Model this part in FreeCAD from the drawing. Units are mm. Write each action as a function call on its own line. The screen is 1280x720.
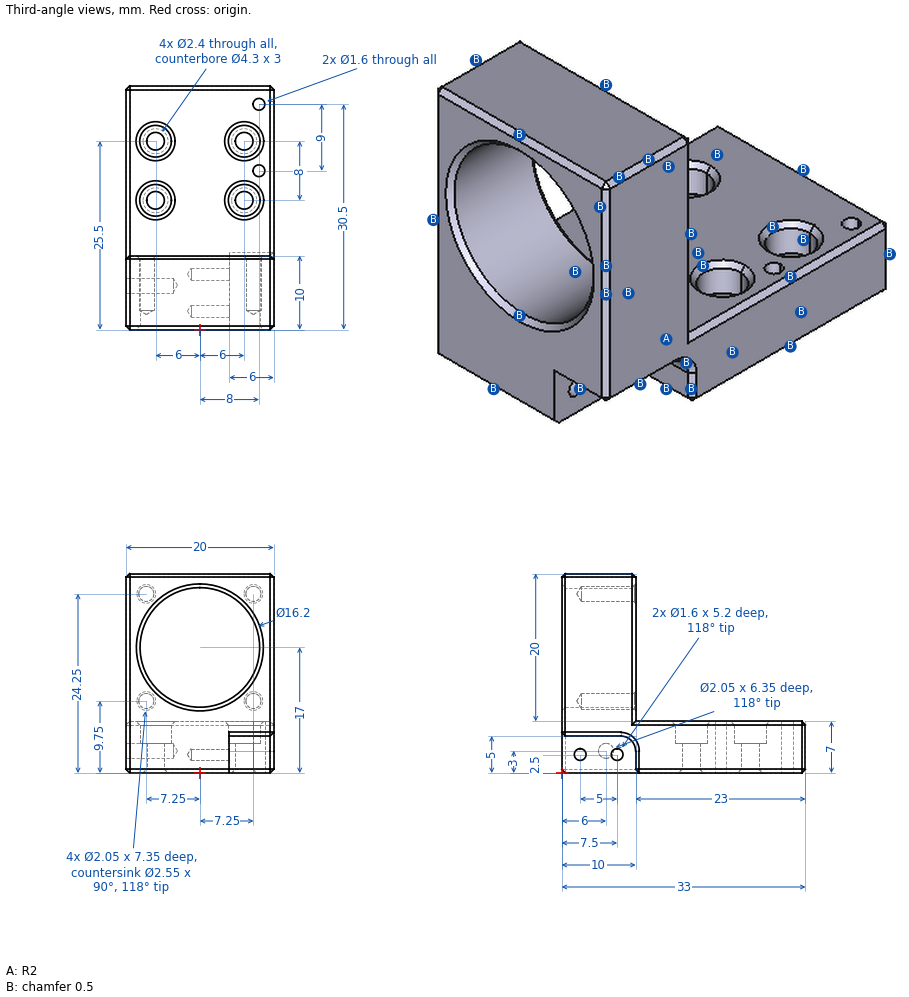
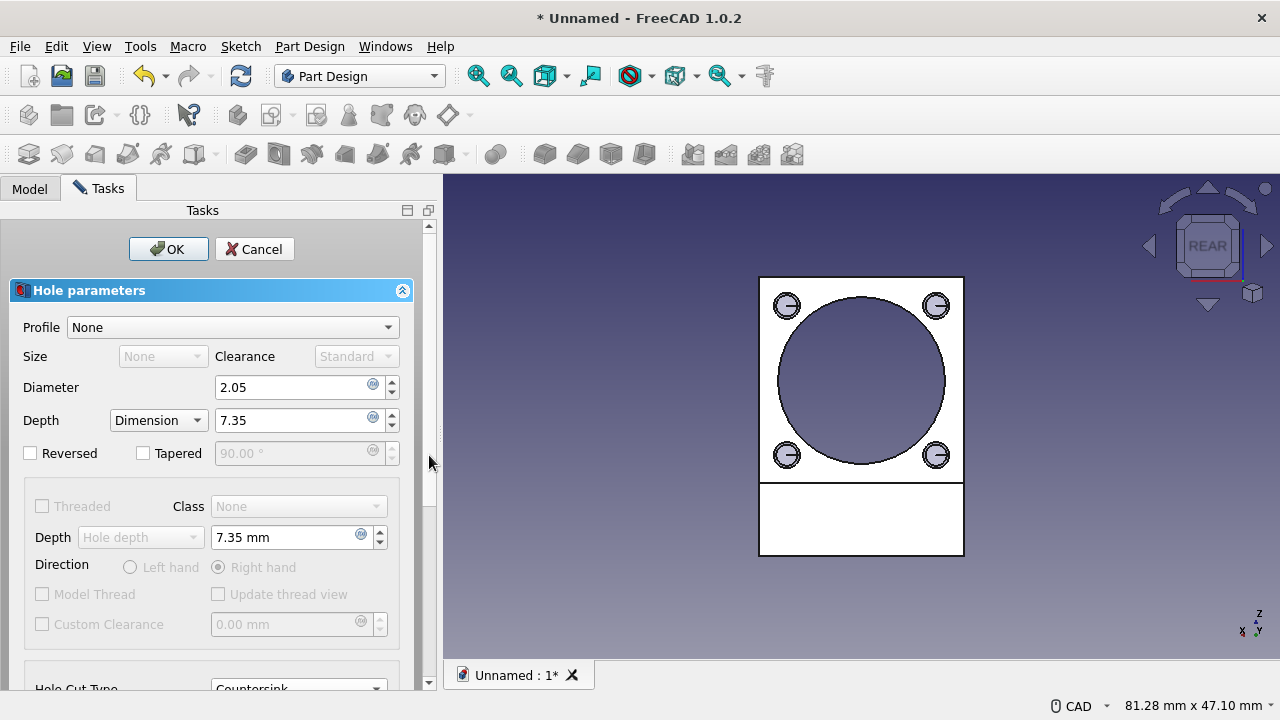
click(169, 249)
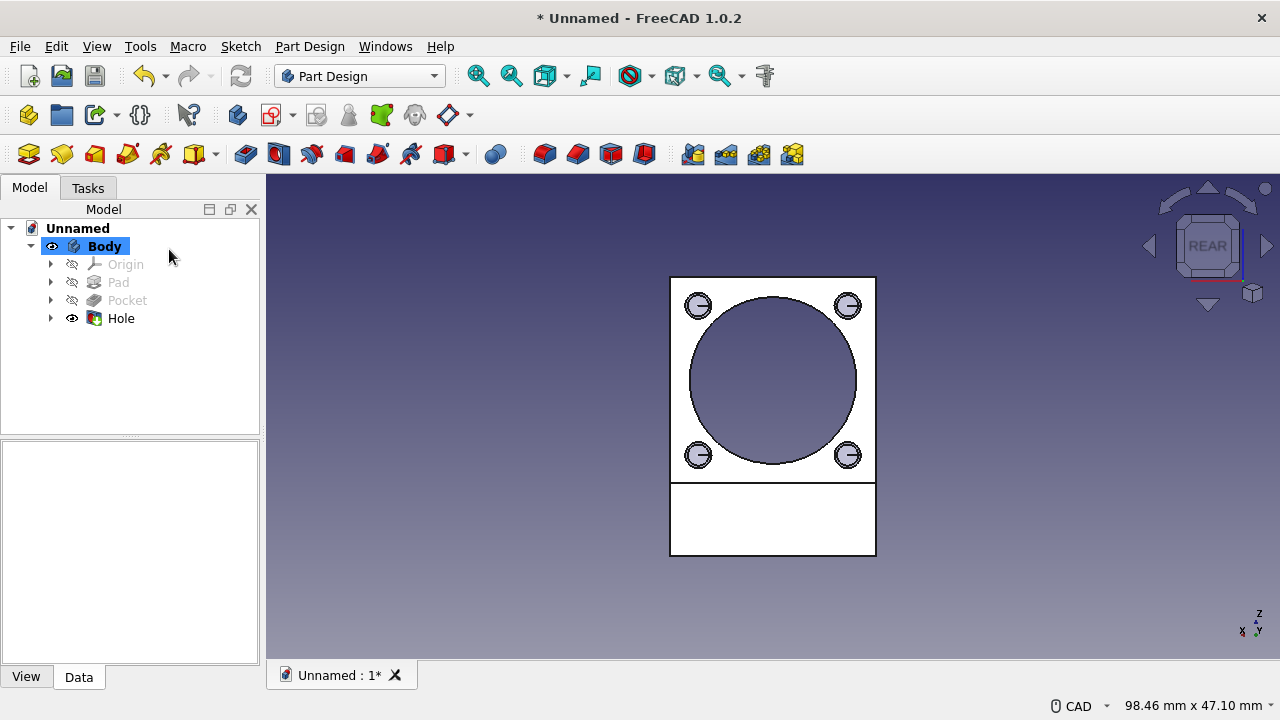
key(0)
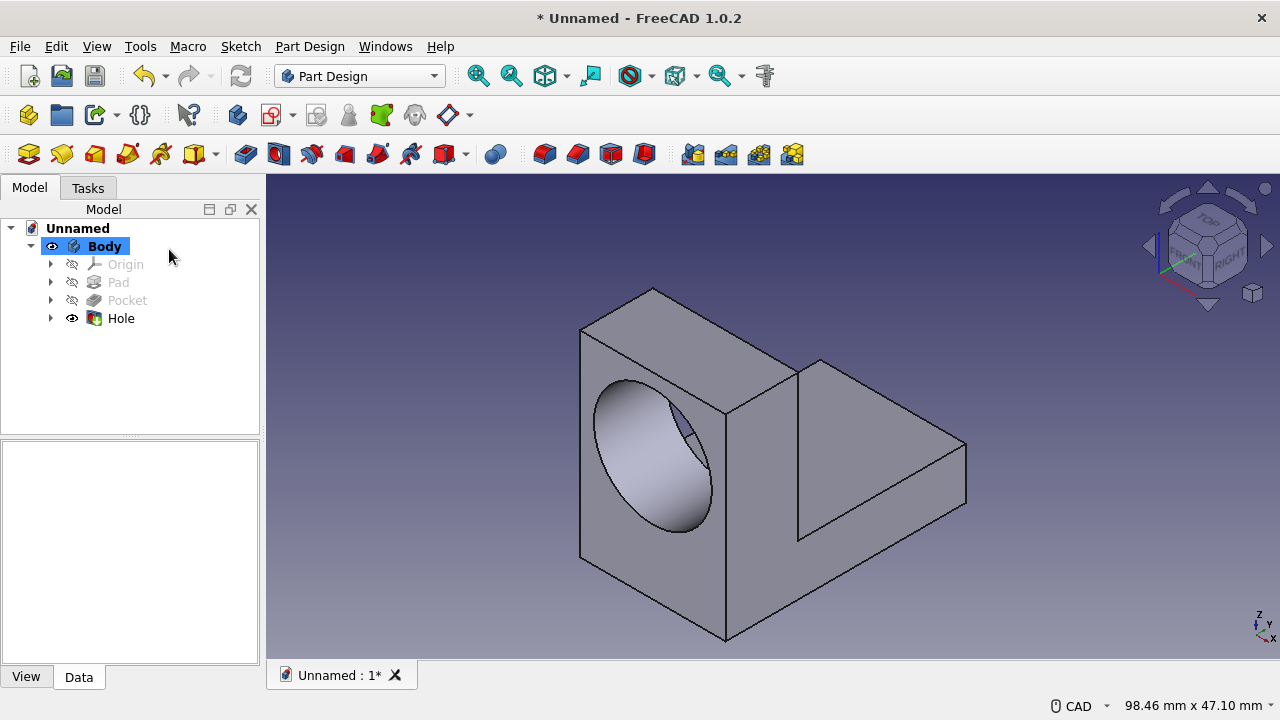
click(809, 449)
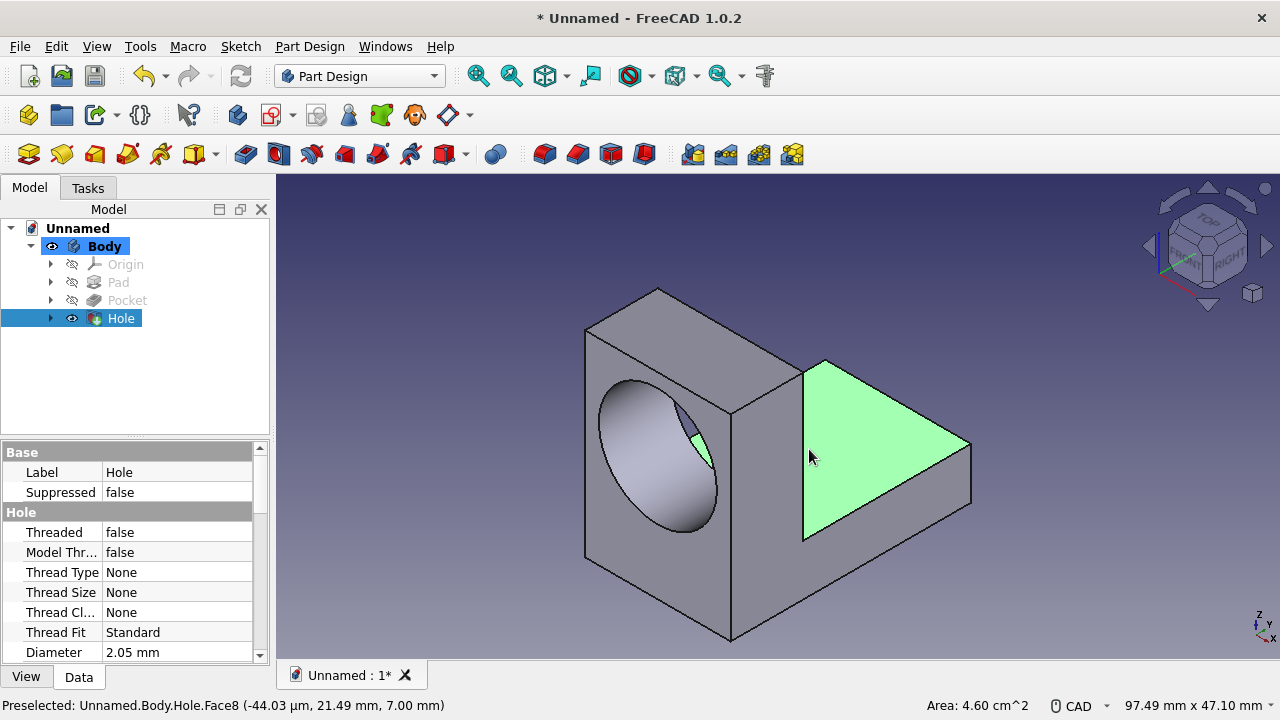
click(270, 116)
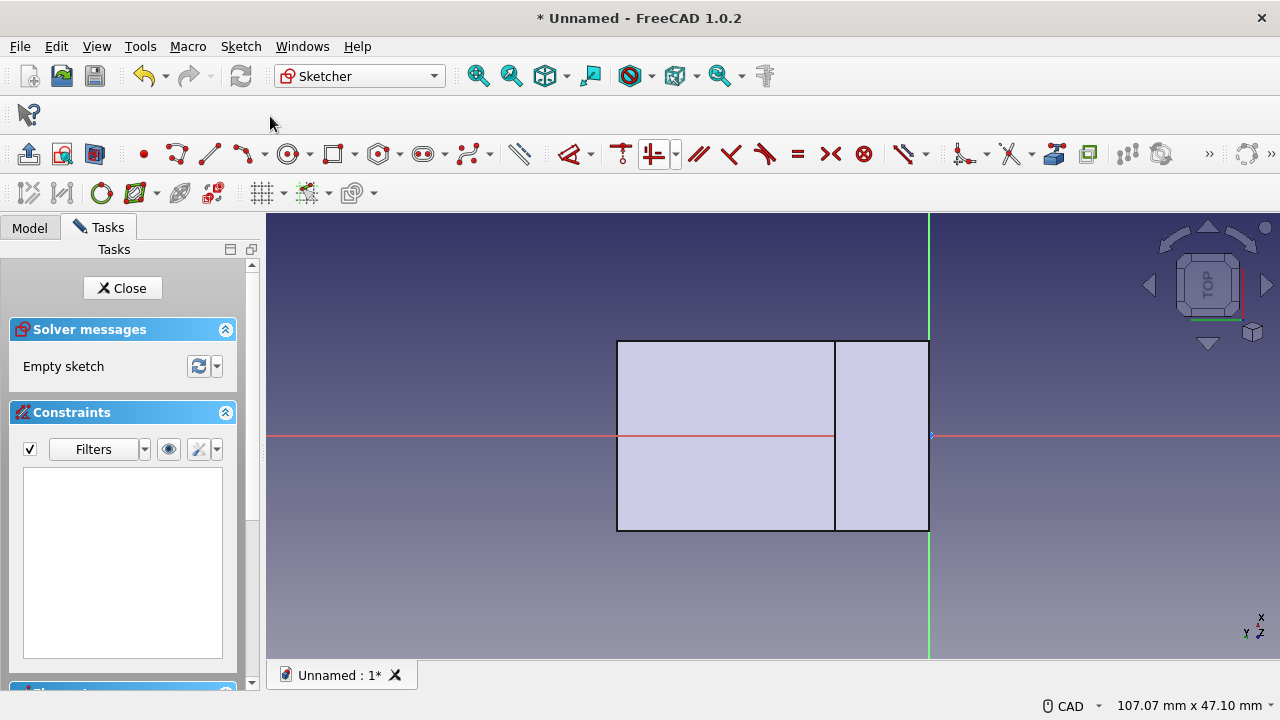
scroll(883, 436, up, 4)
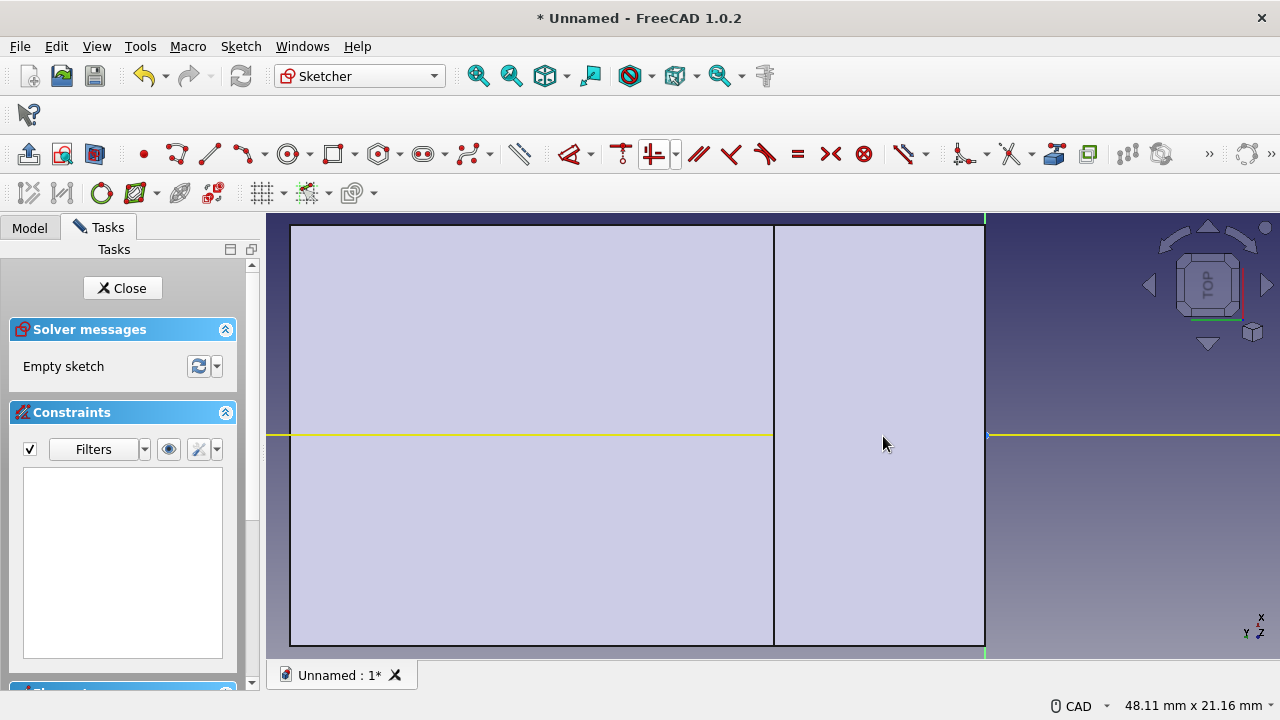
key(g)
key(c)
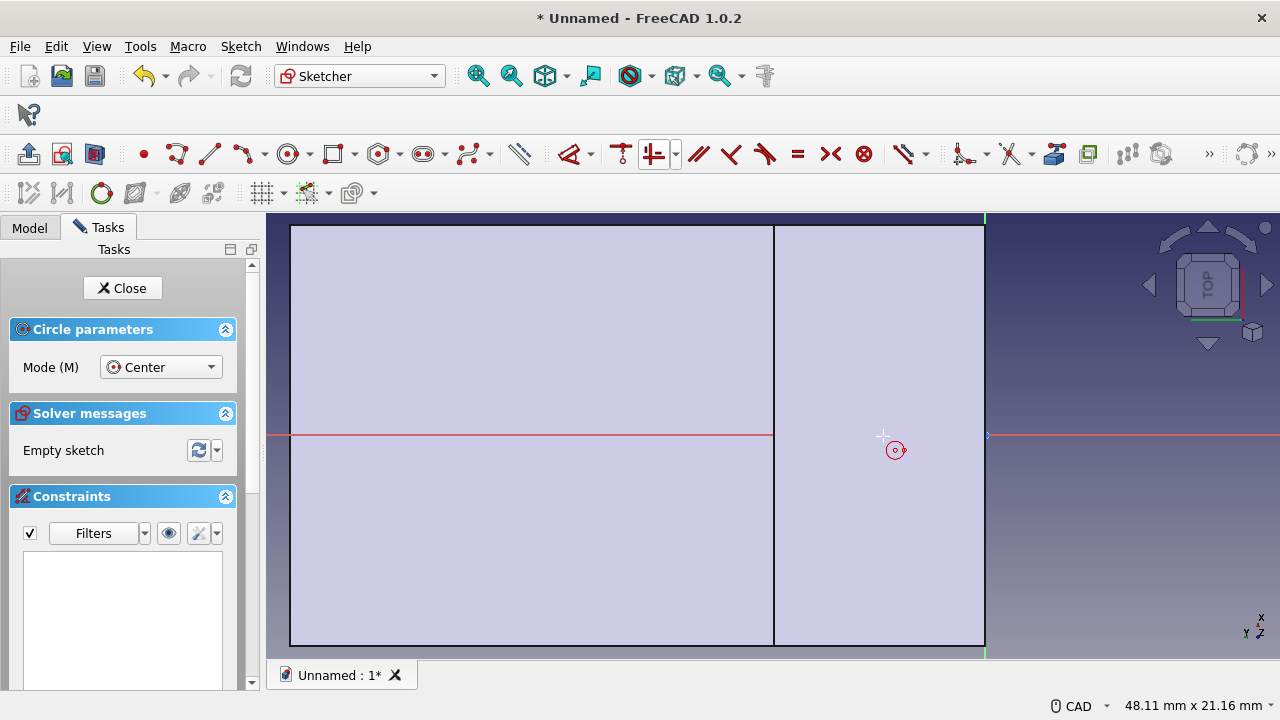
click(448, 562)
move(466, 544)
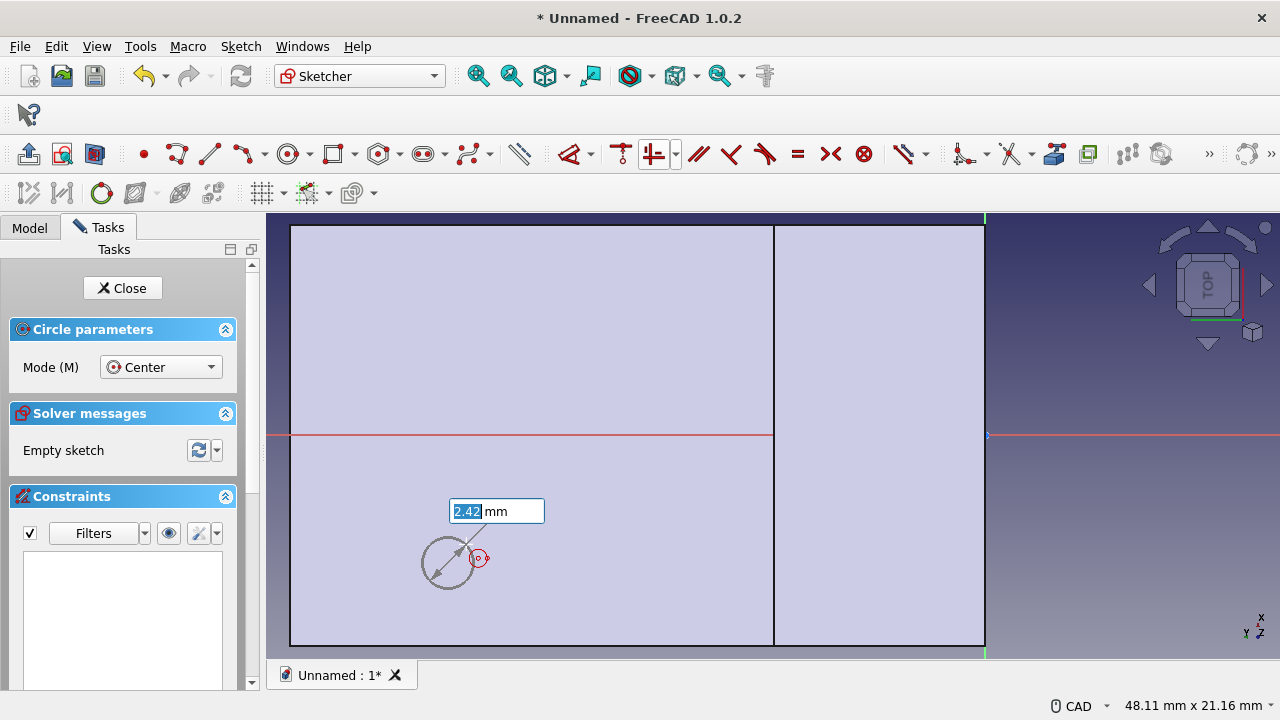
text(2.4)
key(Return)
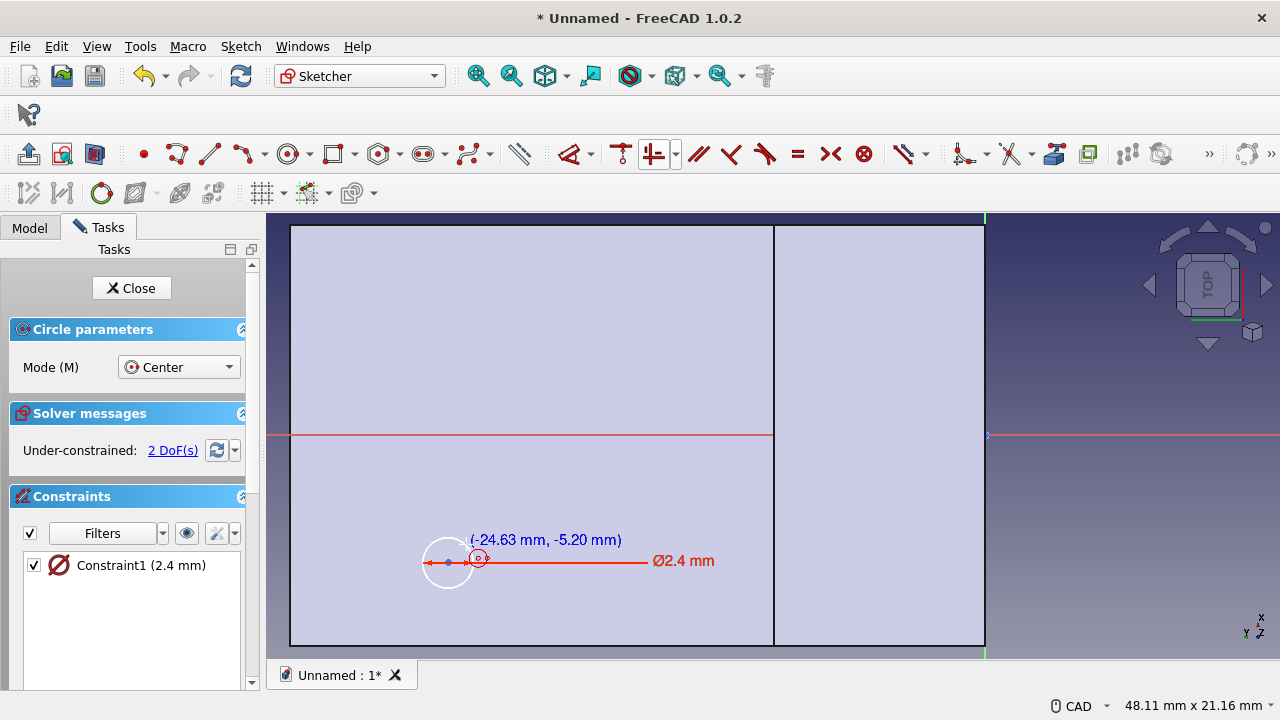
click(448, 309)
move(466, 291)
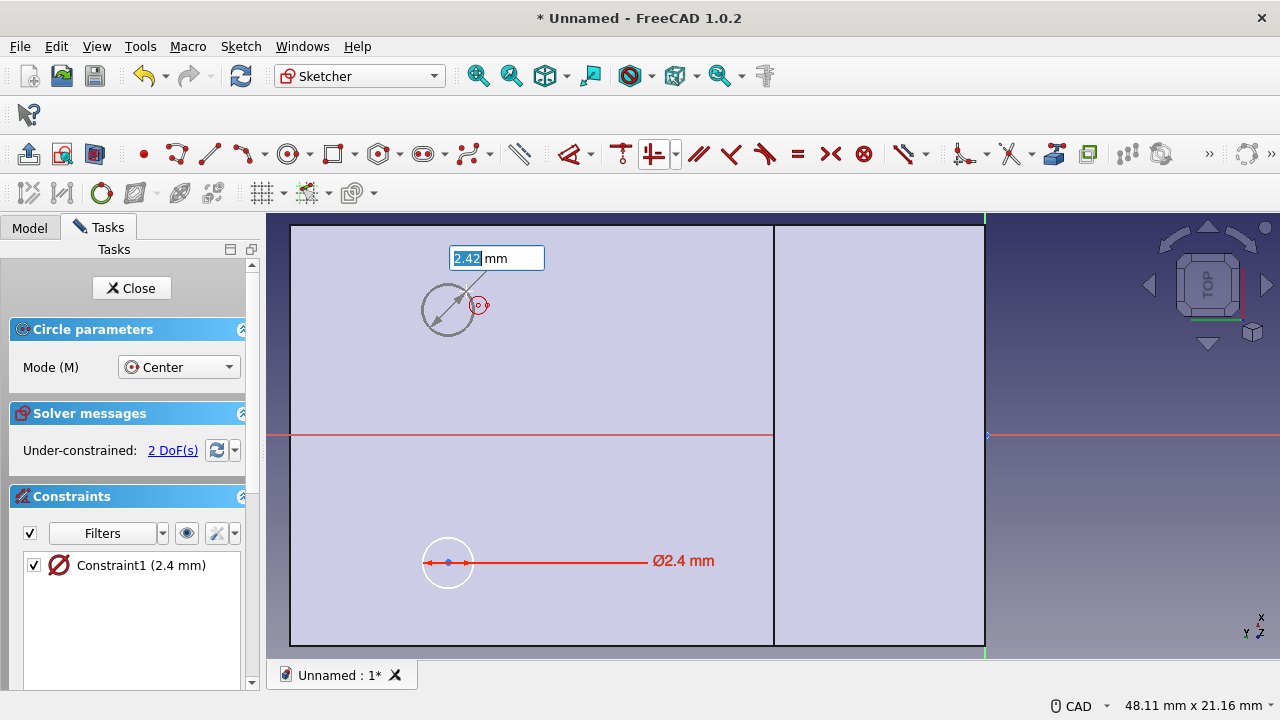
text(2.4)
key(Return)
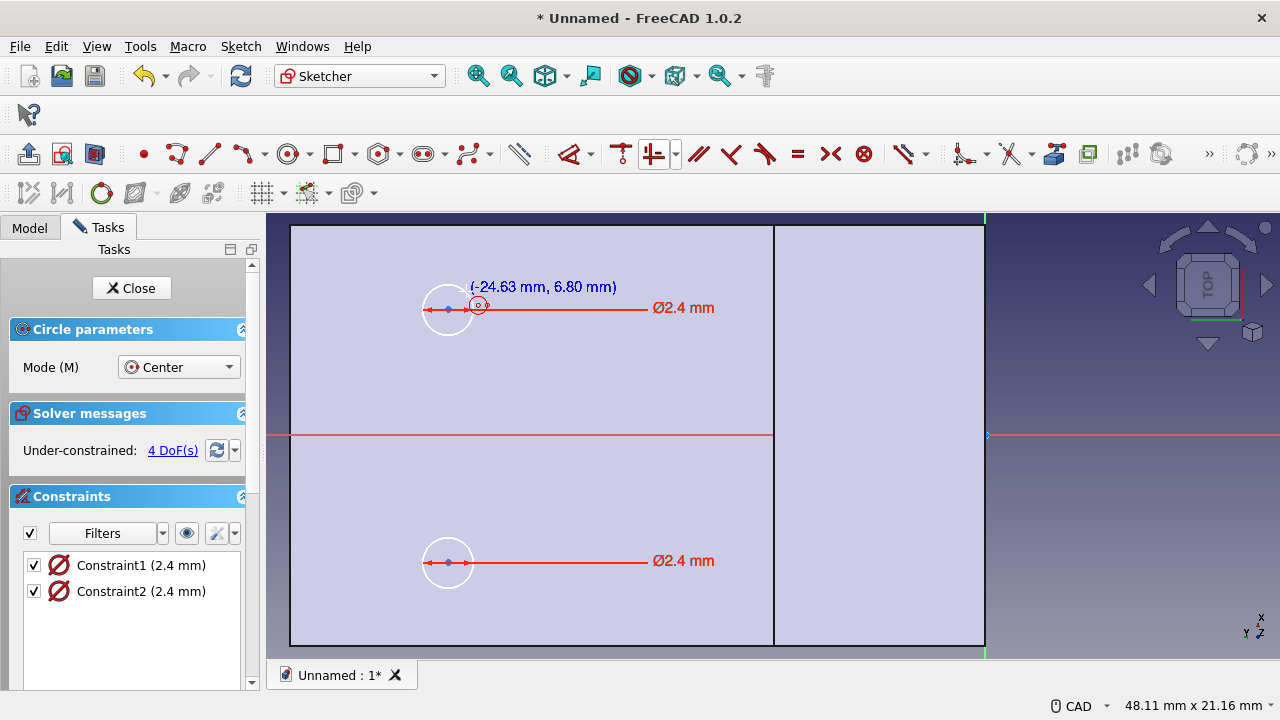
click(616, 309)
move(634, 291)